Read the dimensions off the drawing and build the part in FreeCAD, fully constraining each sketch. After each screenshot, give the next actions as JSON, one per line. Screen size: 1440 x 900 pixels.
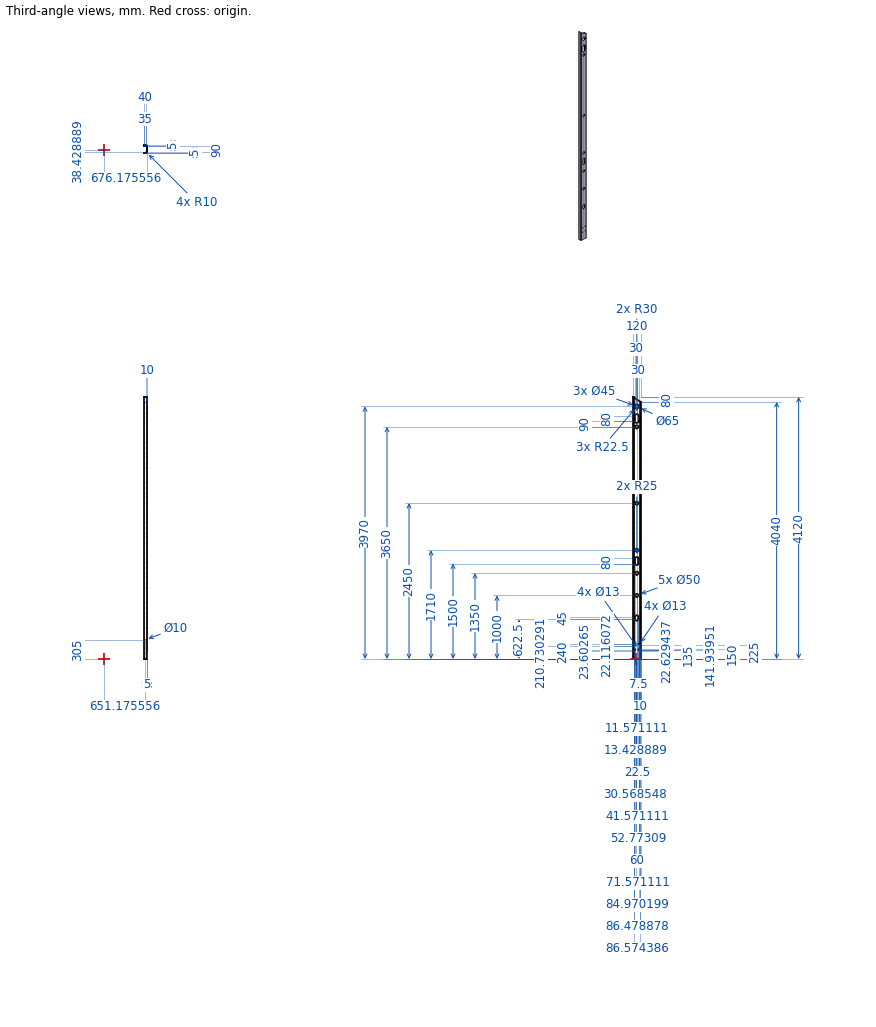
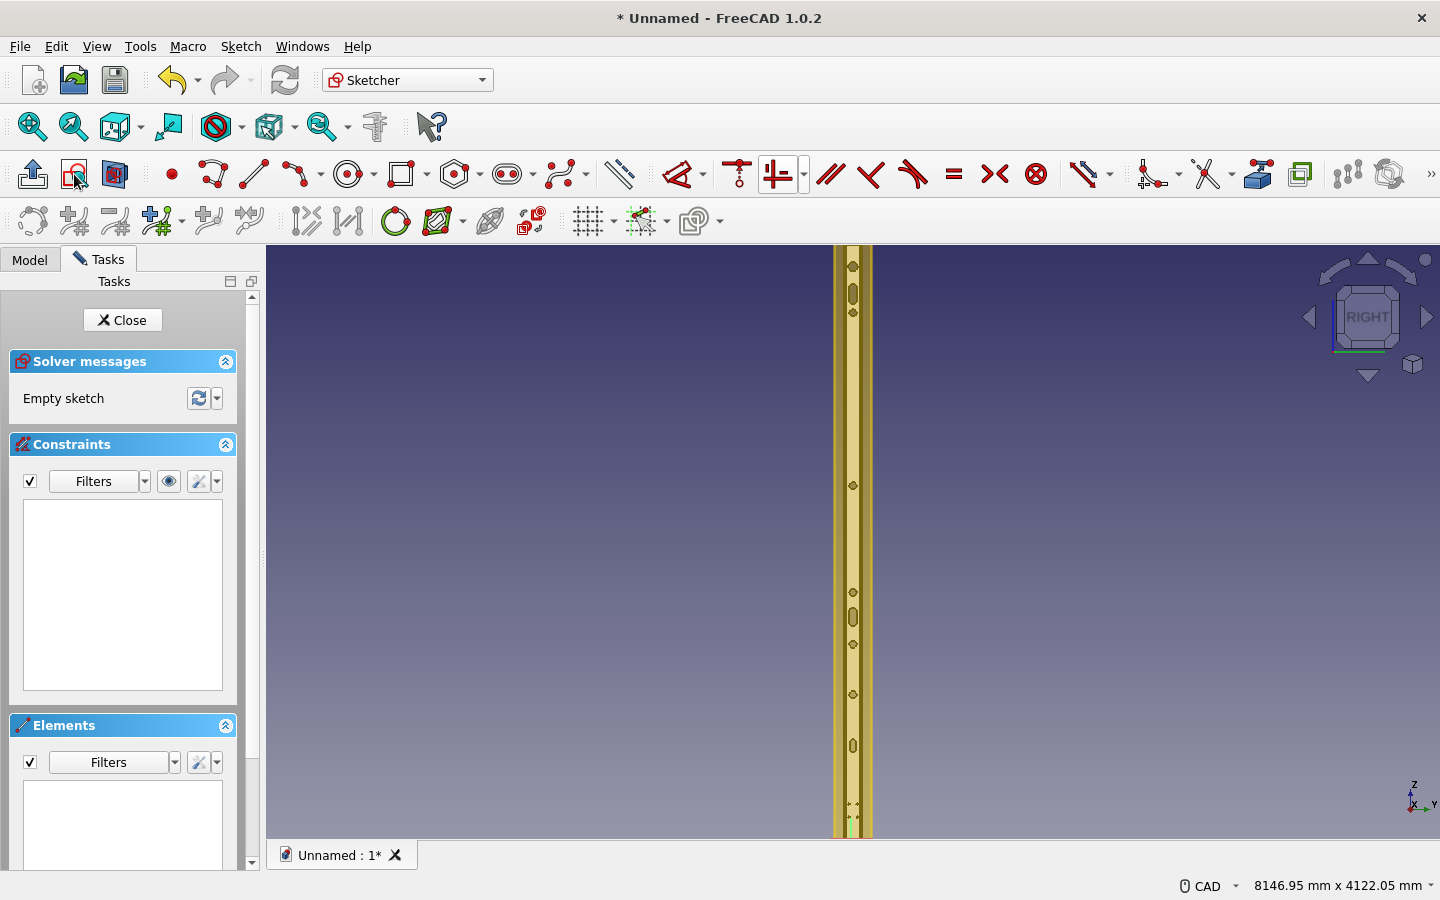
{"action": "scroll", "coordinate": [784, 542], "scroll_direction": "down", "scroll_amount": 5}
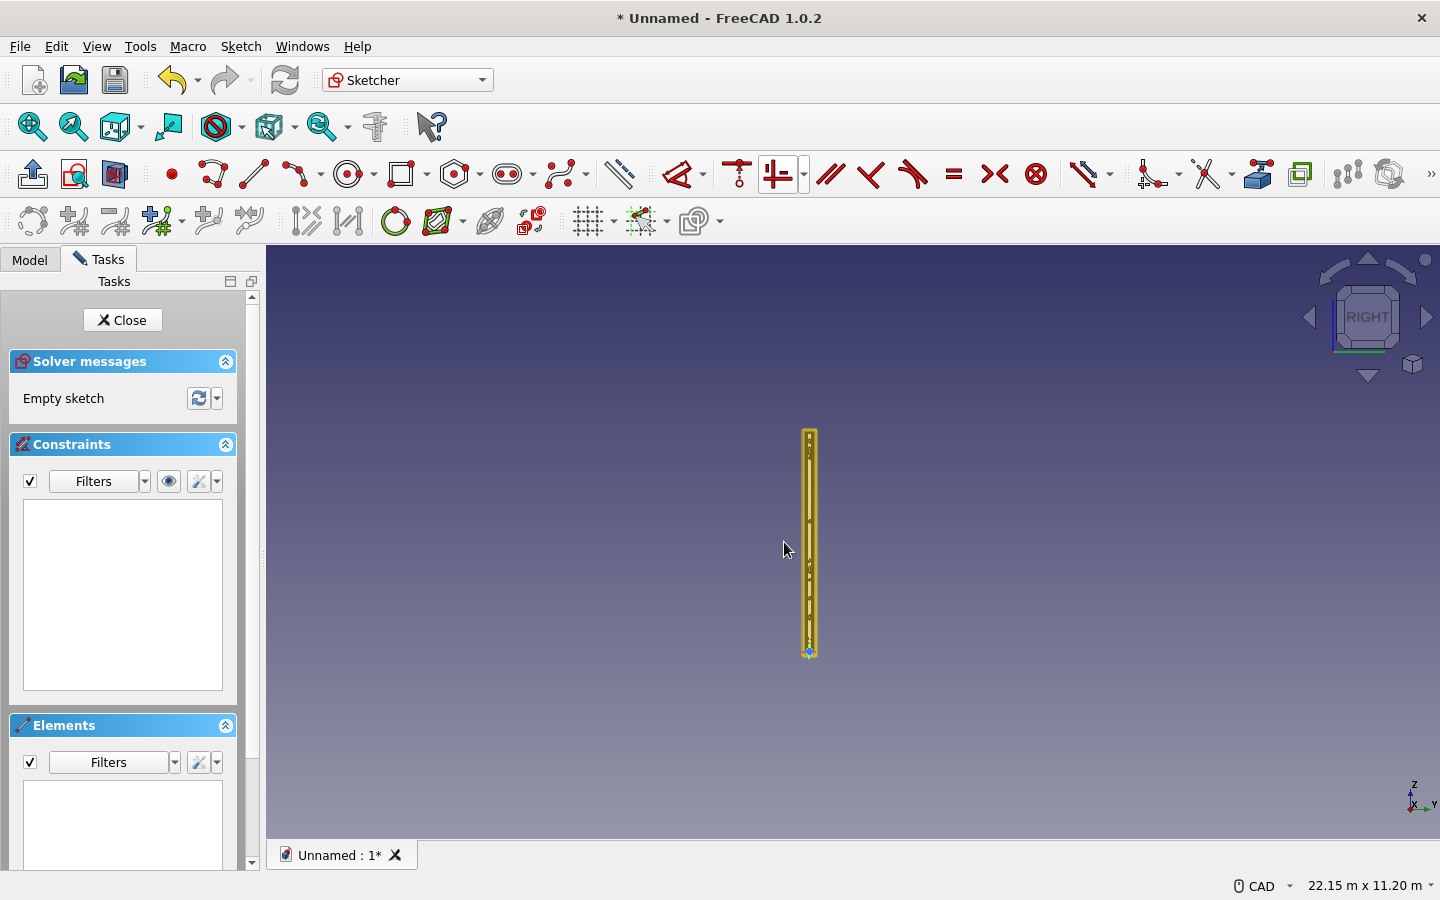
{"action": "scroll", "coordinate": [811, 430], "scroll_direction": "up", "scroll_amount": 15}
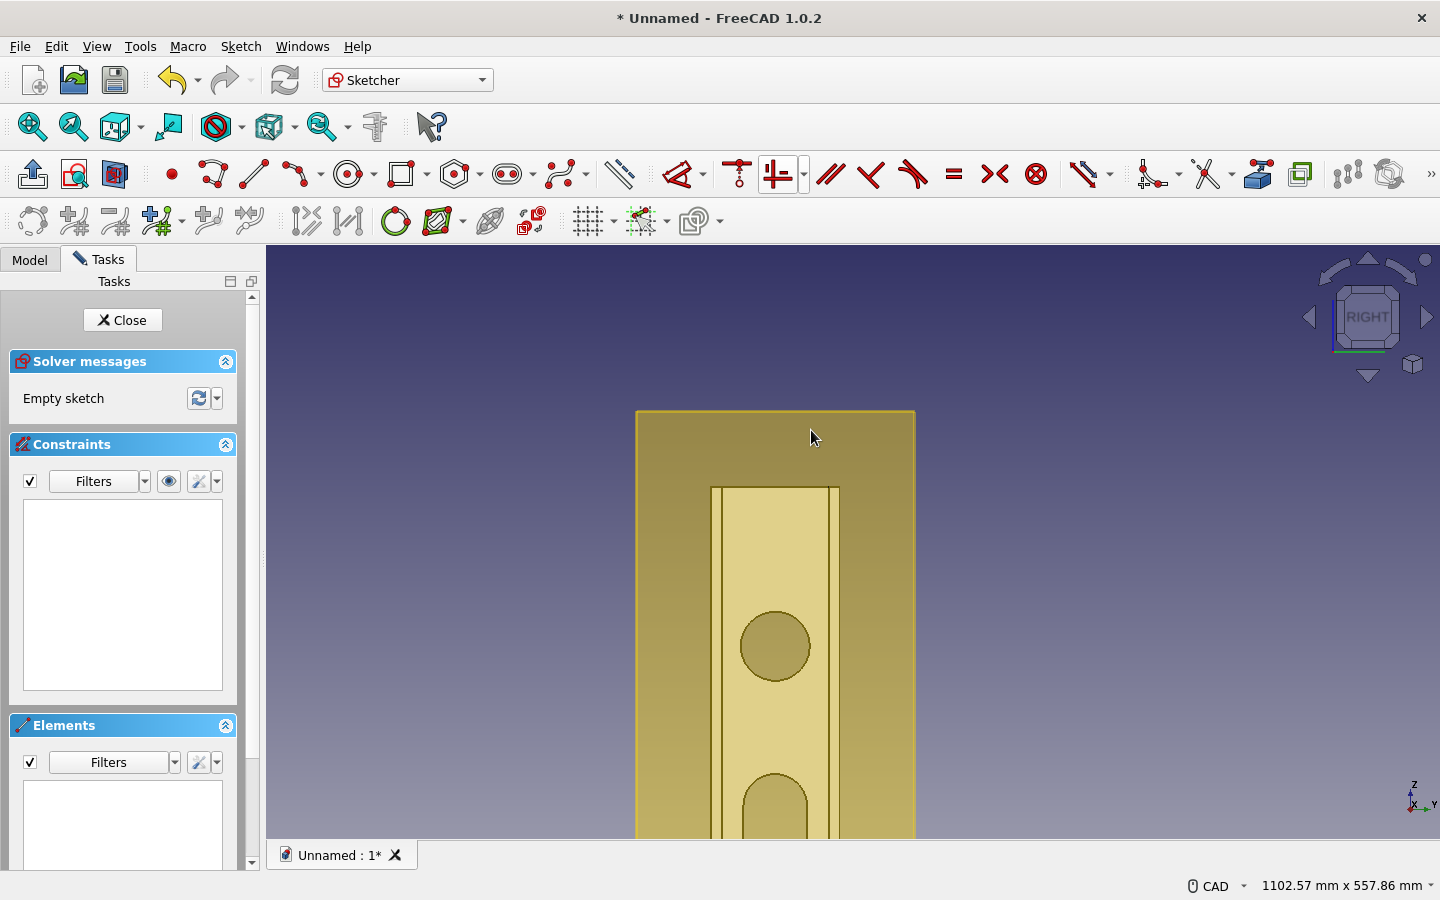
{"action": "scroll", "coordinate": [772, 525], "scroll_direction": "up", "scroll_amount": 7}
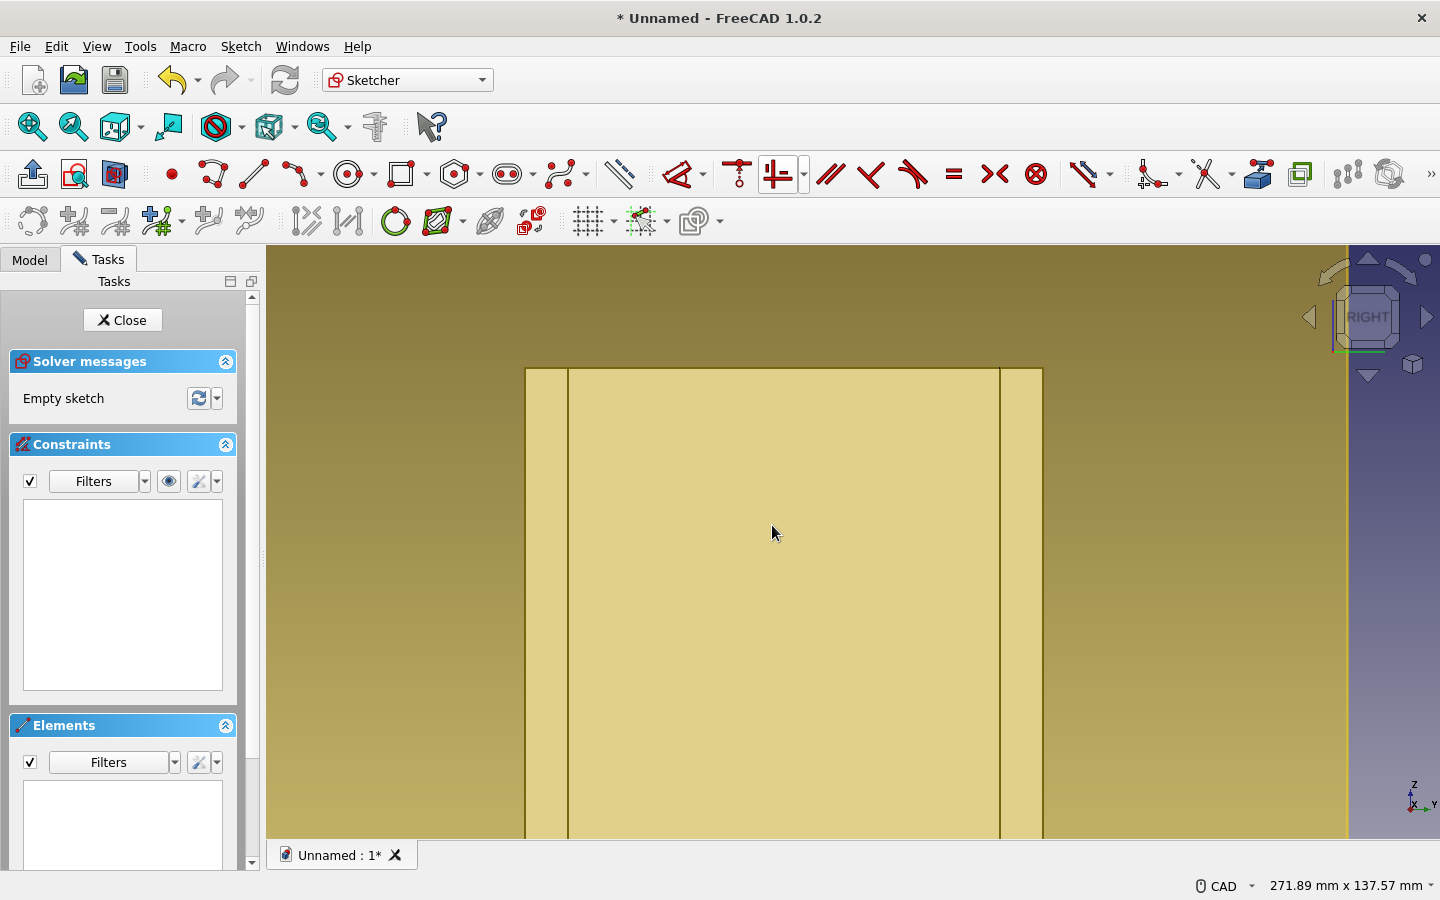
{"action": "key", "text": "g m"}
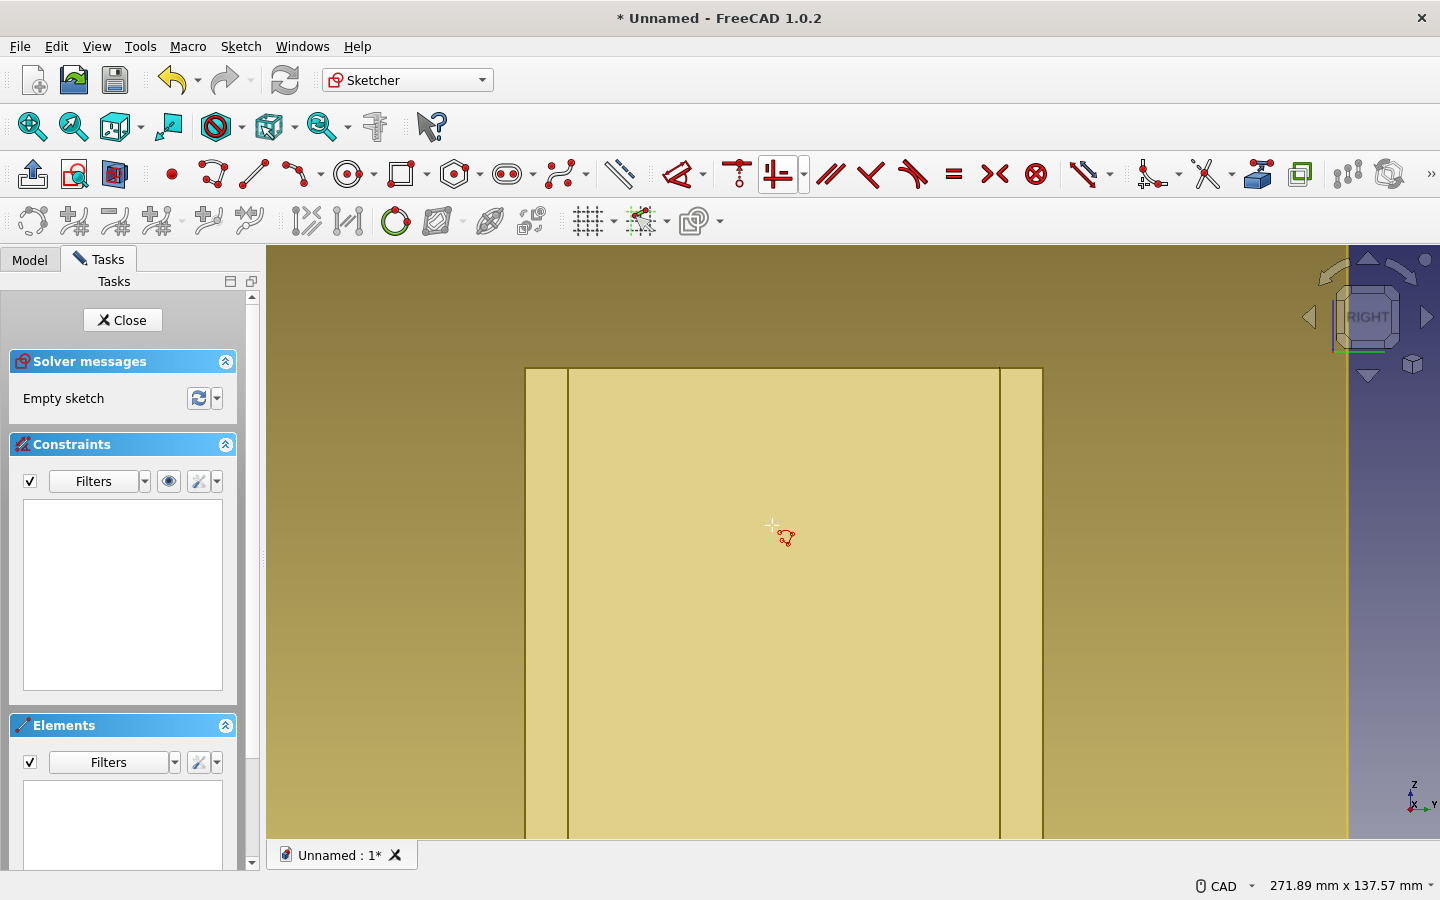
{"action": "left_click", "coordinate": [1043, 713]}
{"action": "left_click", "coordinate": [1043, 368]}
{"action": "left_click", "coordinate": [525, 368]}
{"action": "left_click", "coordinate": [1043, 714]}
{"action": "key", "text": "Escape"}
{"action": "key", "text": "Escape"}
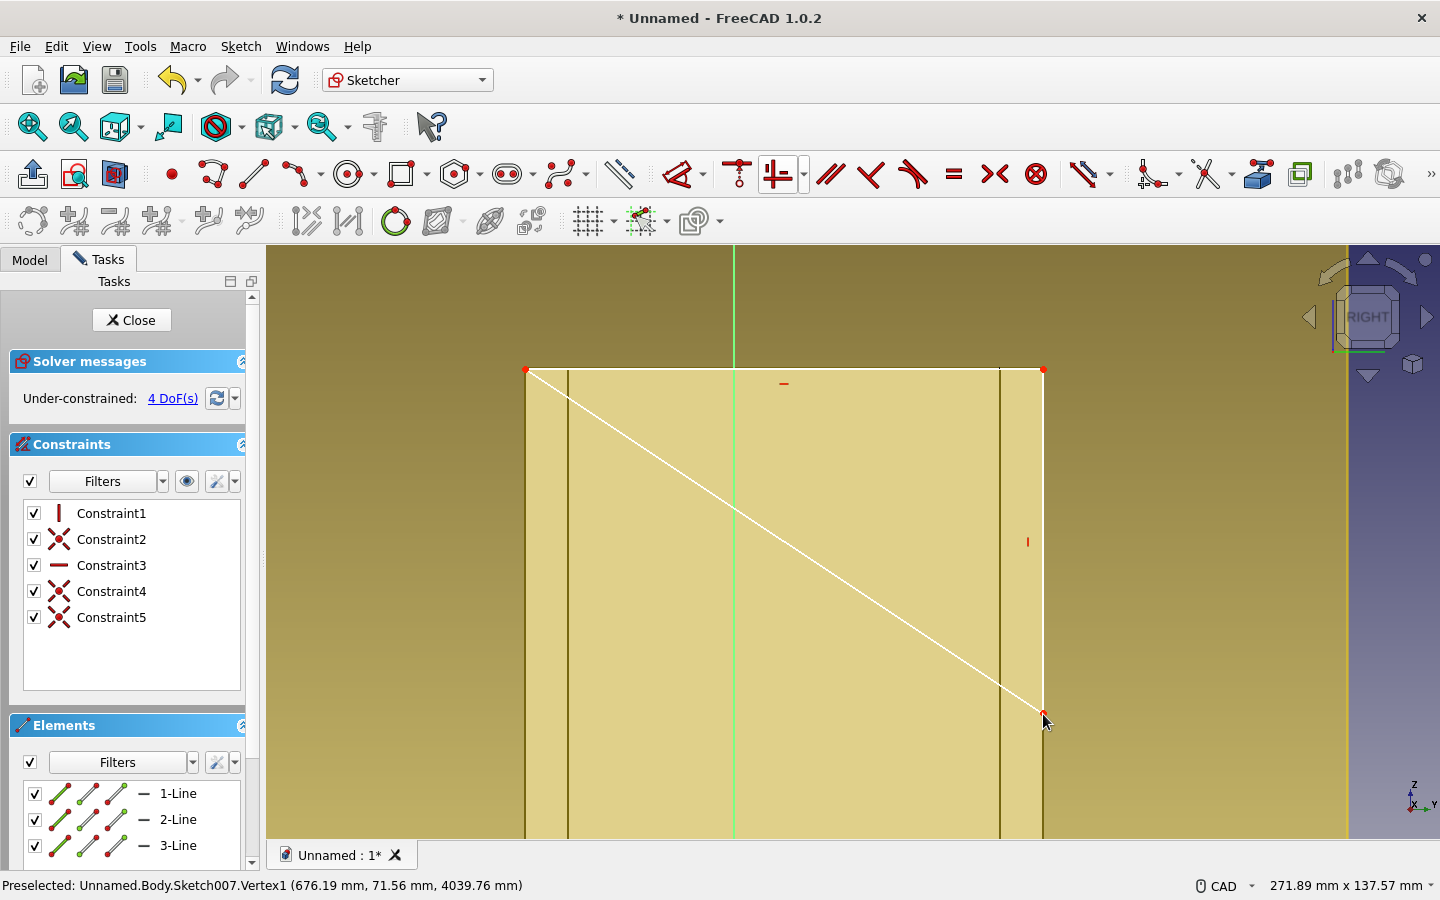
{"action": "key", "text": "d"}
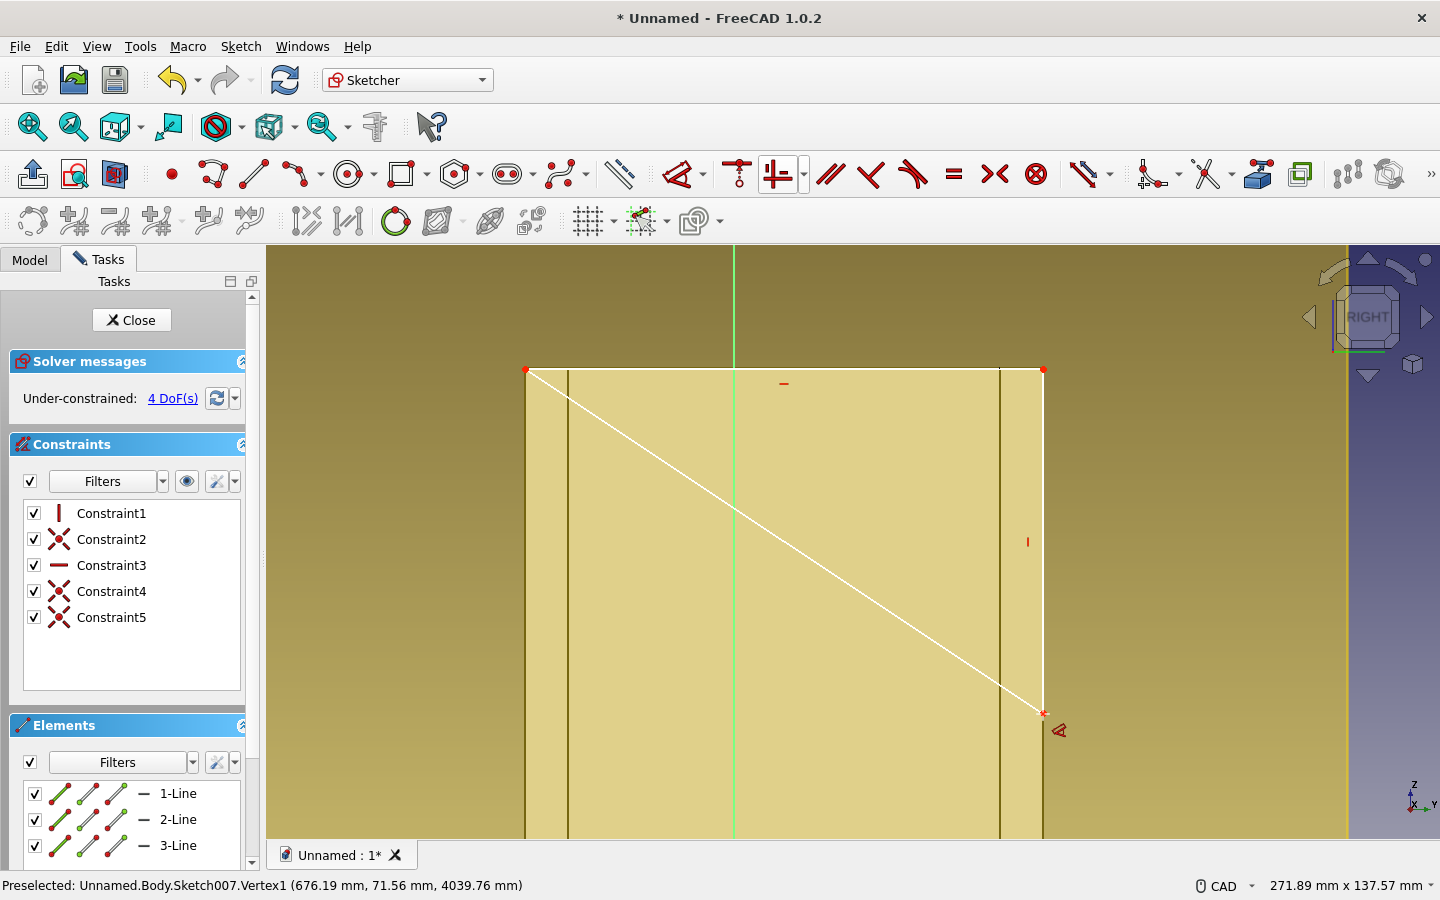
{"action": "left_click", "coordinate": [1043, 611]}
{"action": "left_click", "coordinate": [1077, 542]}